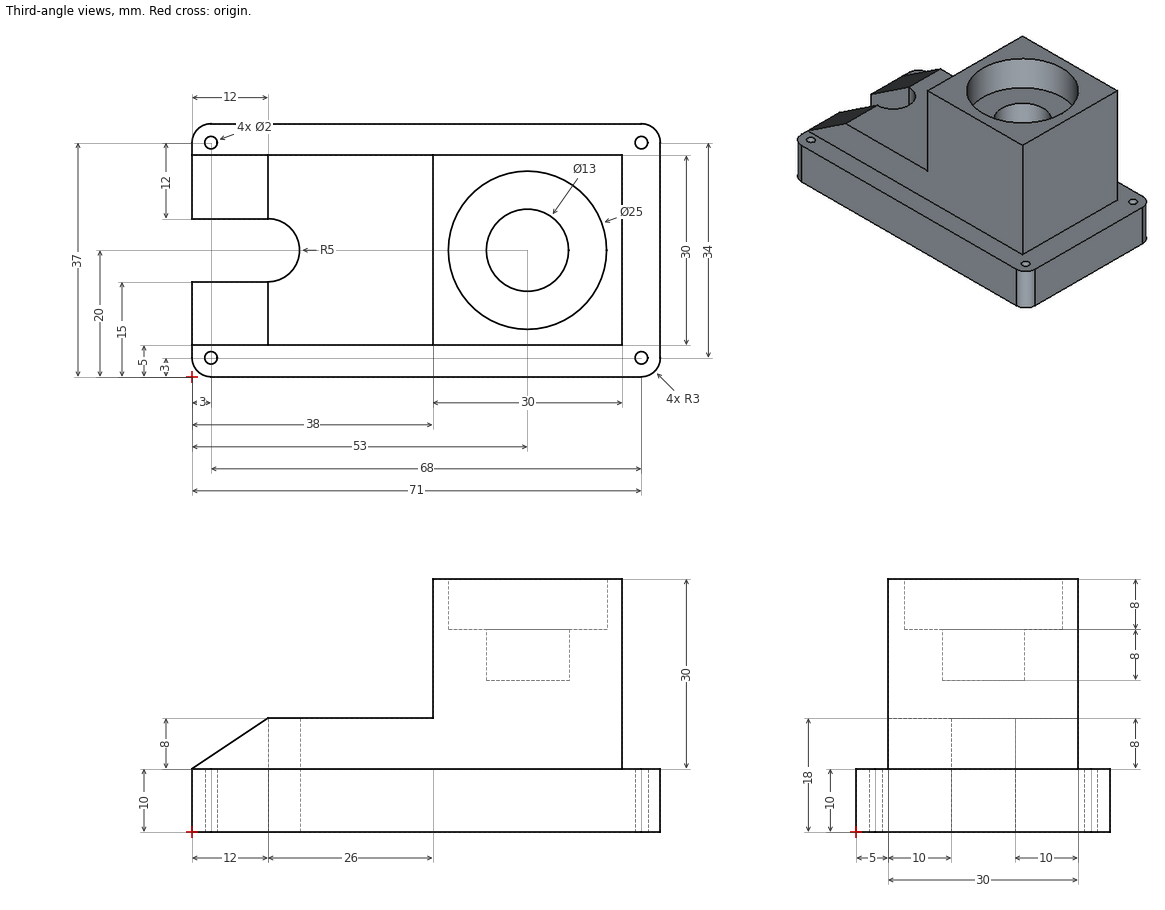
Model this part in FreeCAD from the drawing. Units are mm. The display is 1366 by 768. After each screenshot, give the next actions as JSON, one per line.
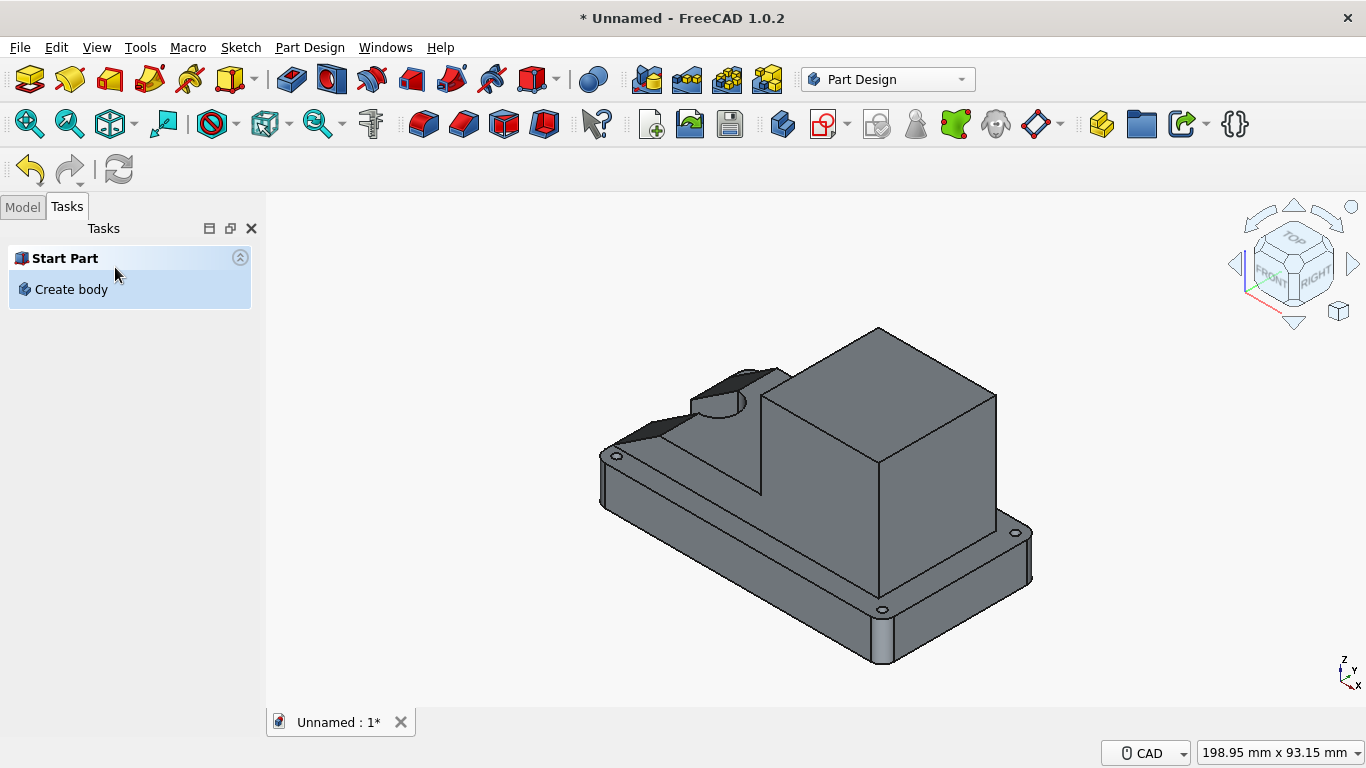
{"action": "left_click", "coordinate": [879, 394]}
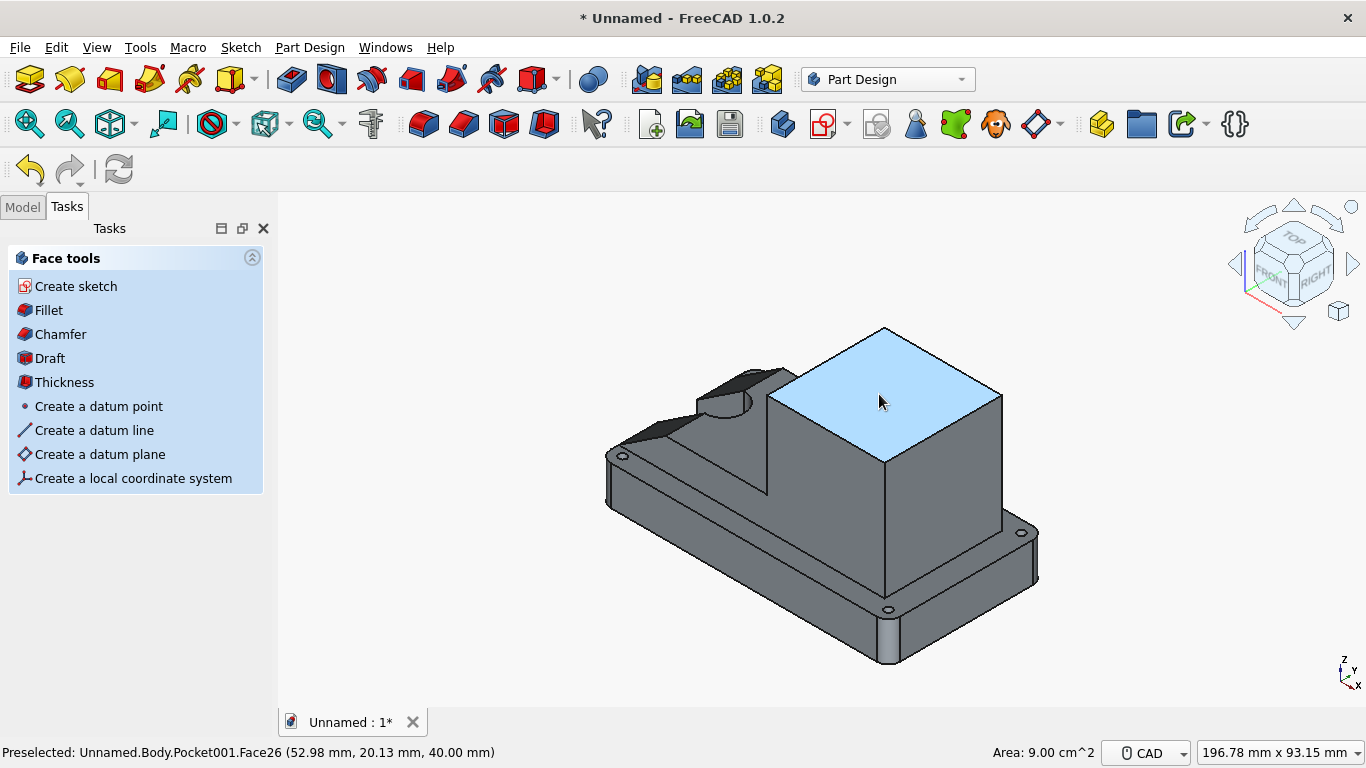
{"action": "left_click", "coordinate": [824, 124]}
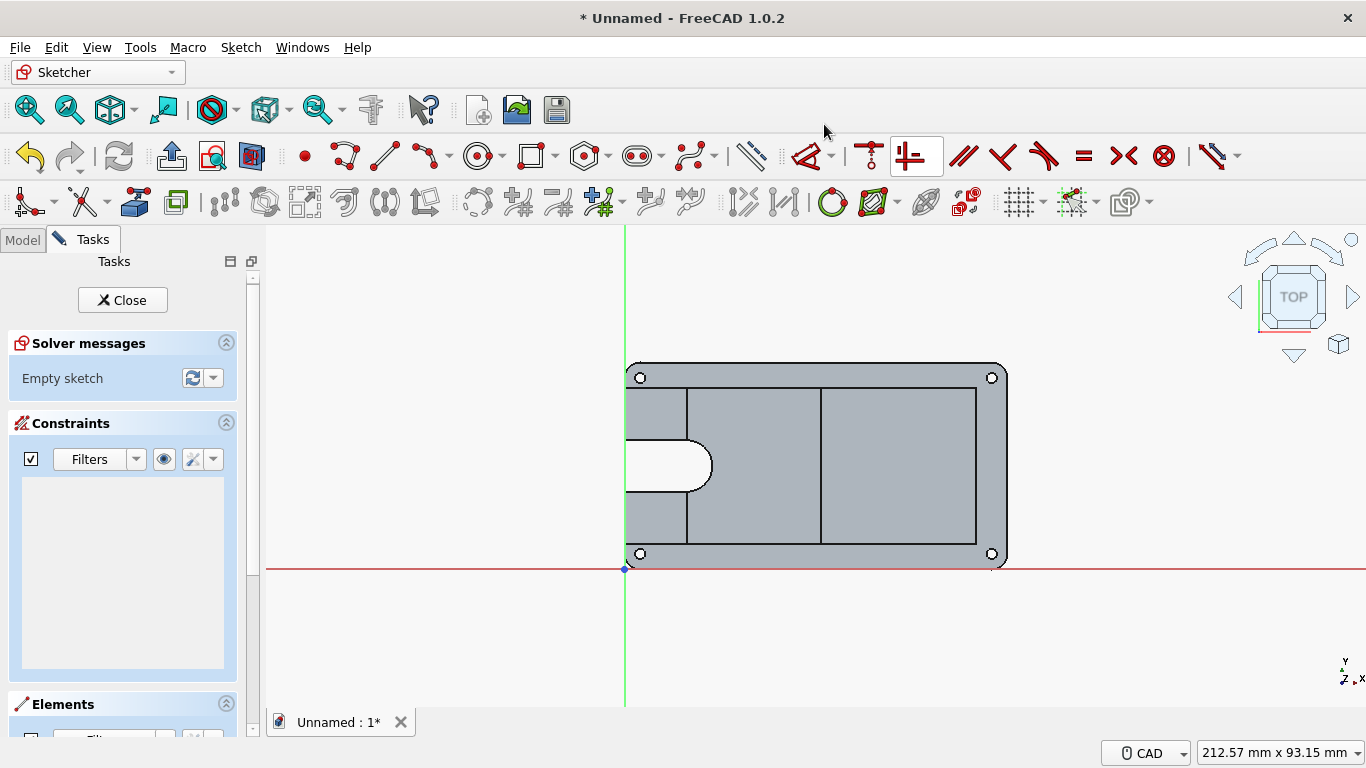
{"action": "scroll", "coordinate": [1022, 466], "scroll_direction": "up", "scroll_amount": 4}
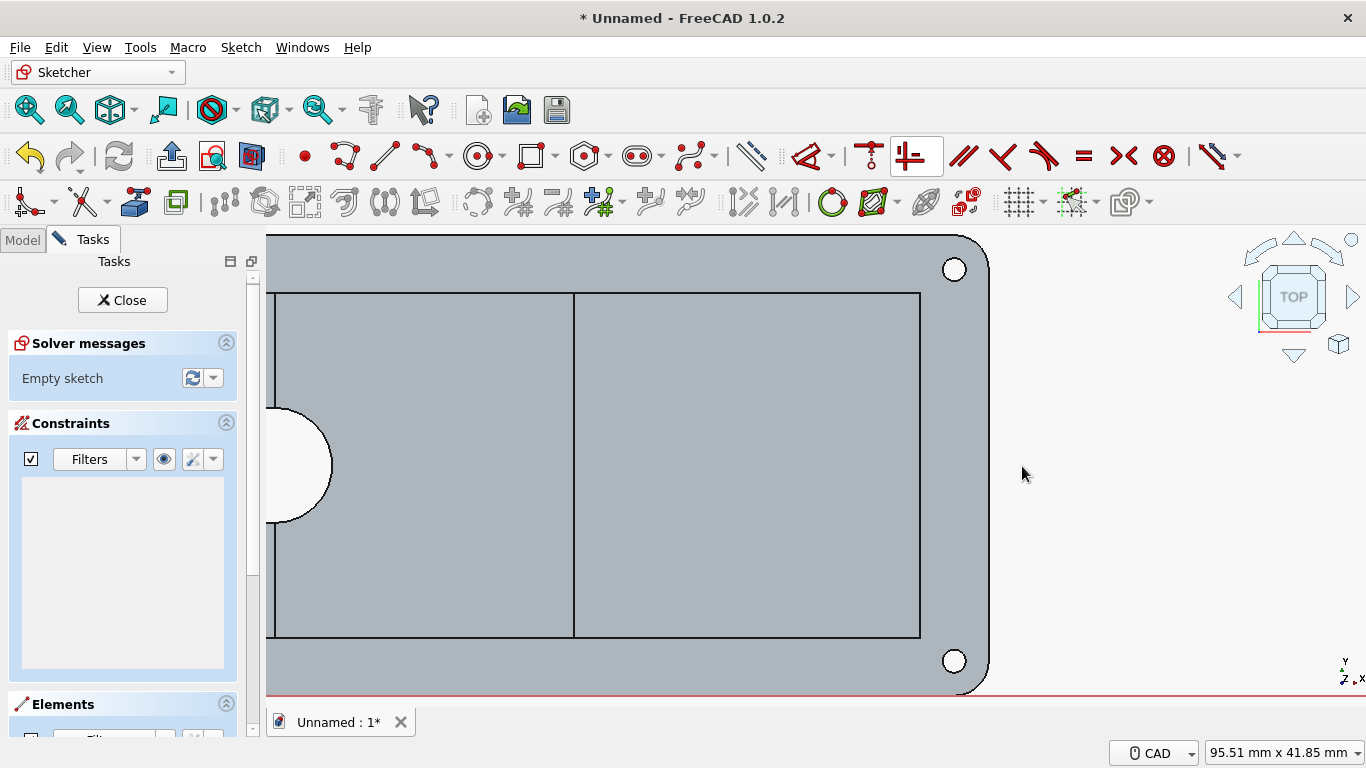
{"action": "left_click", "coordinate": [478, 156]}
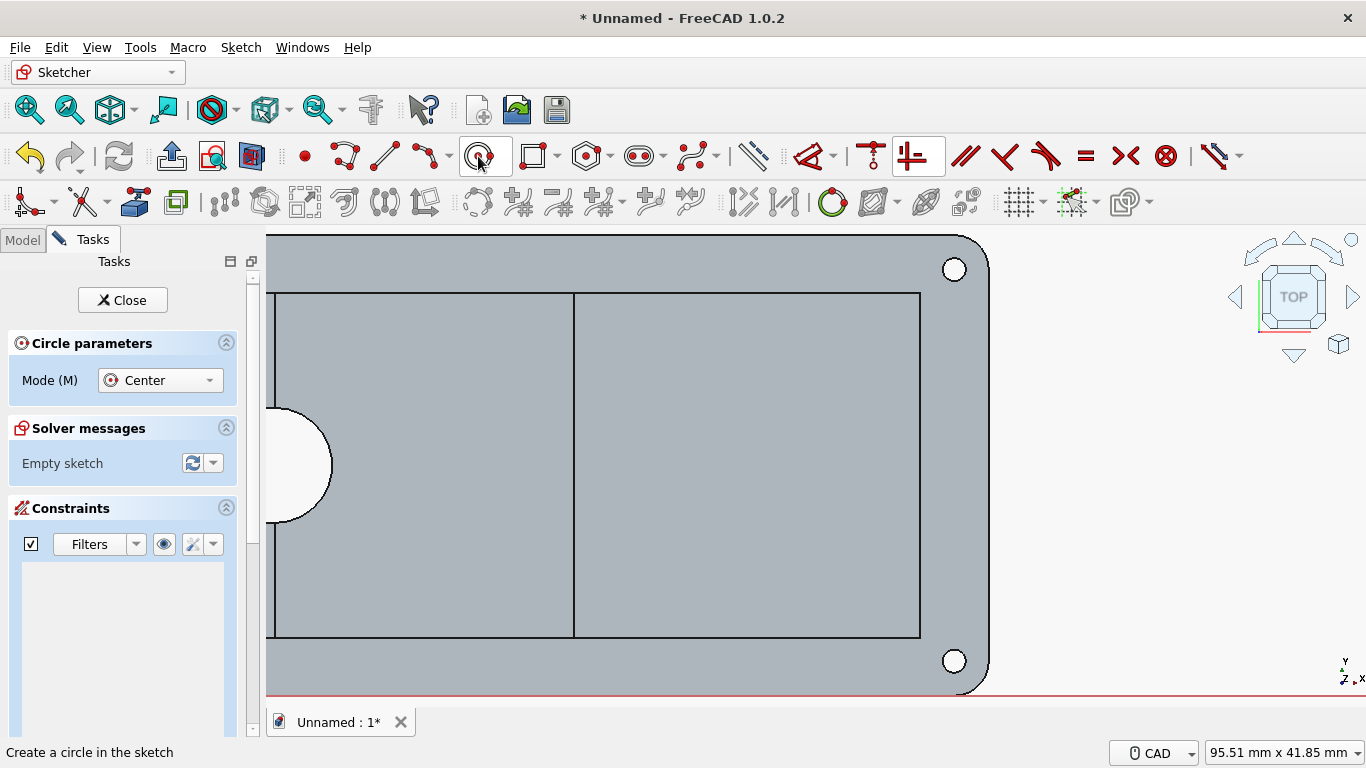
{"action": "left_click", "coordinate": [747, 465]}
{"action": "left_click", "coordinate": [849, 364]}
{"action": "key", "text": "Escape"}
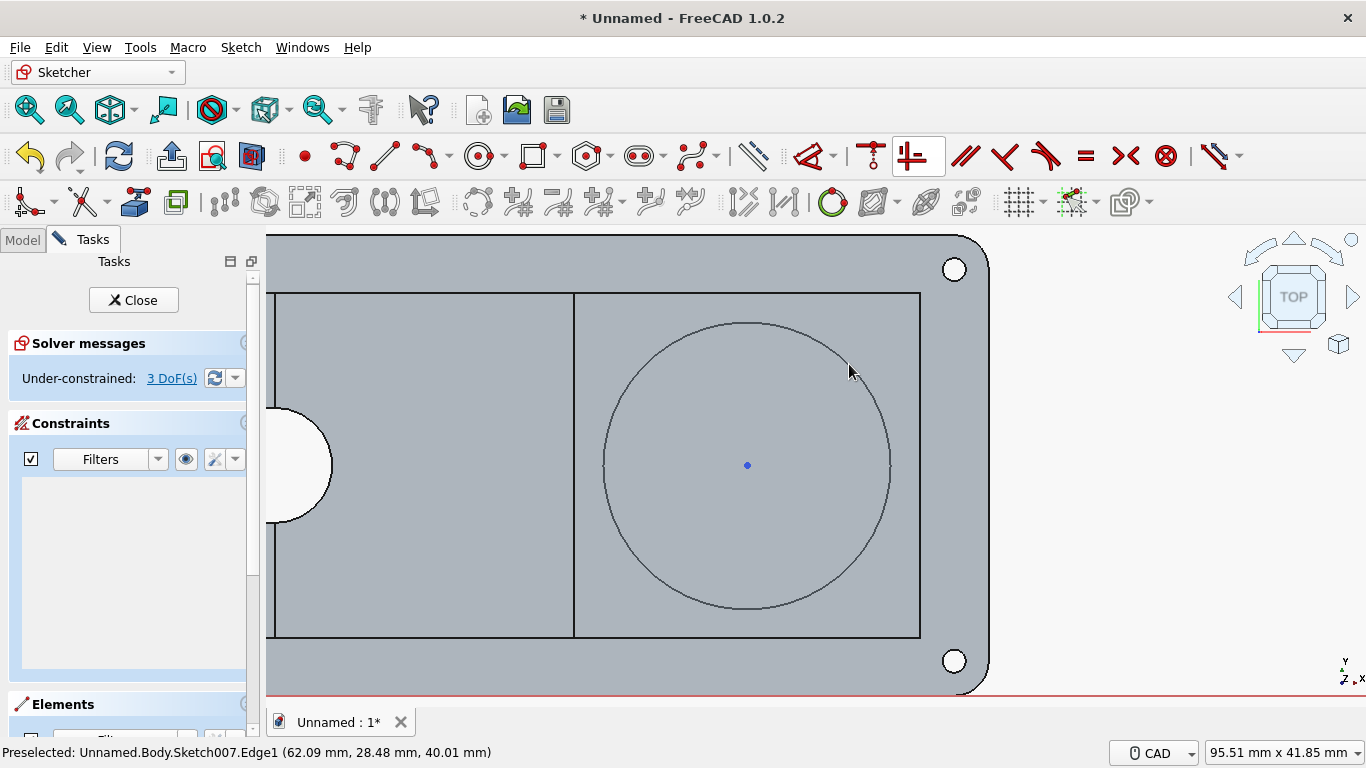
{"action": "left_click", "coordinate": [808, 156]}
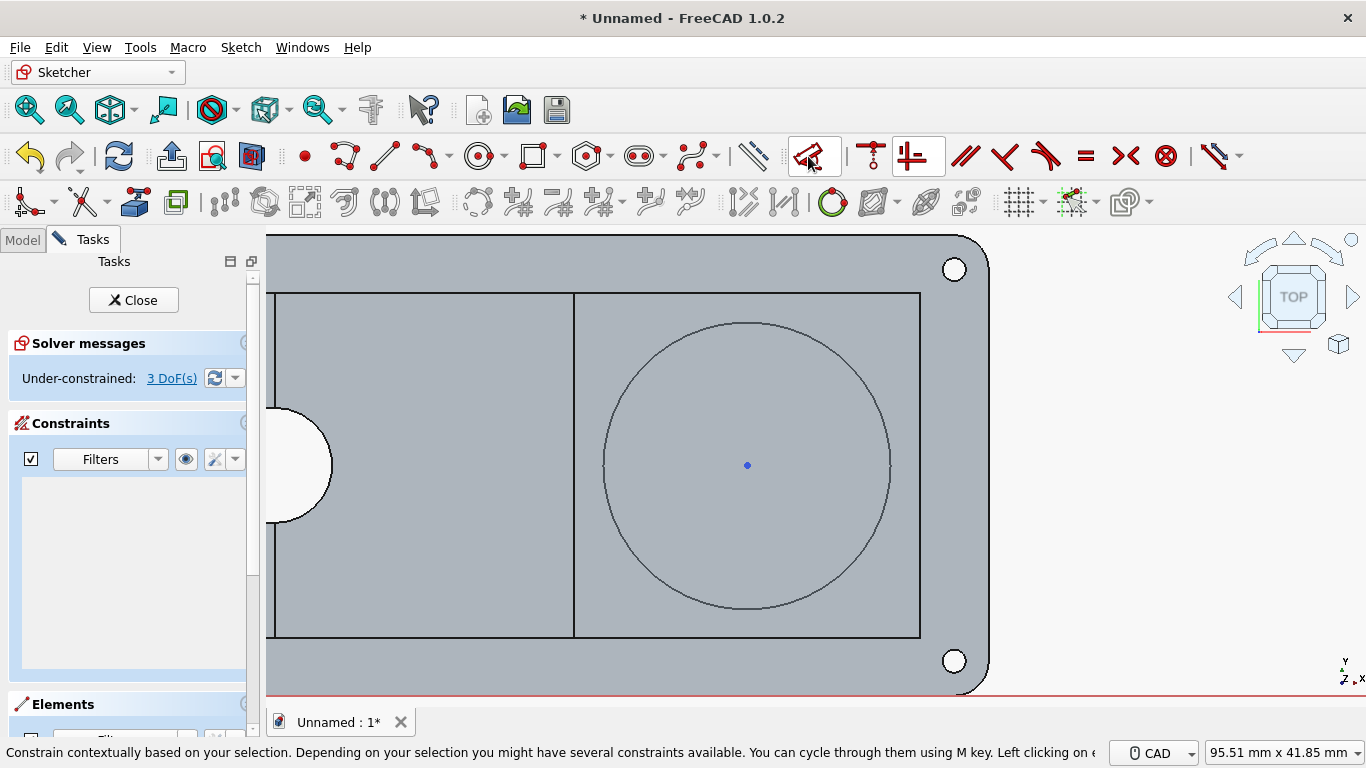
{"action": "left_click", "coordinate": [848, 364]}
{"action": "left_click", "coordinate": [871, 341]}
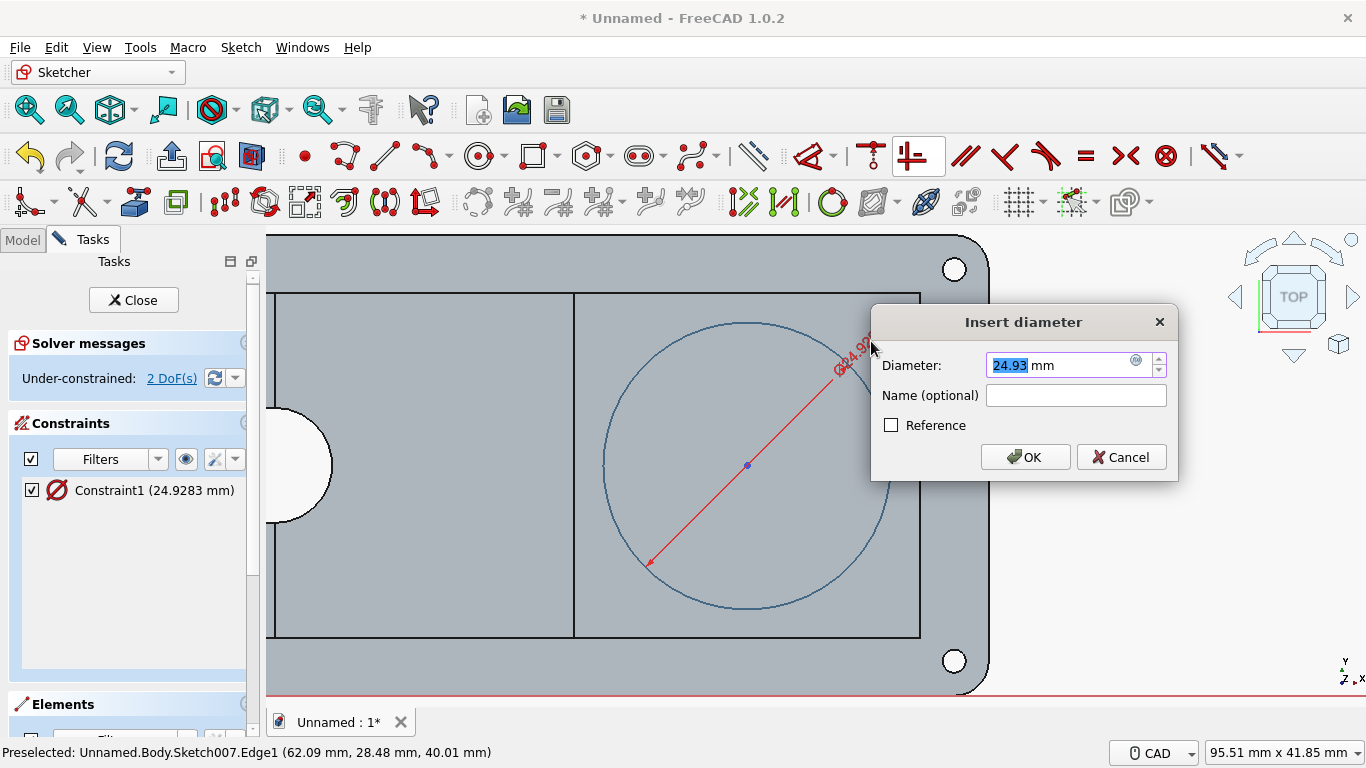
{"action": "type", "text": "25"}
{"action": "key", "text": "Return"}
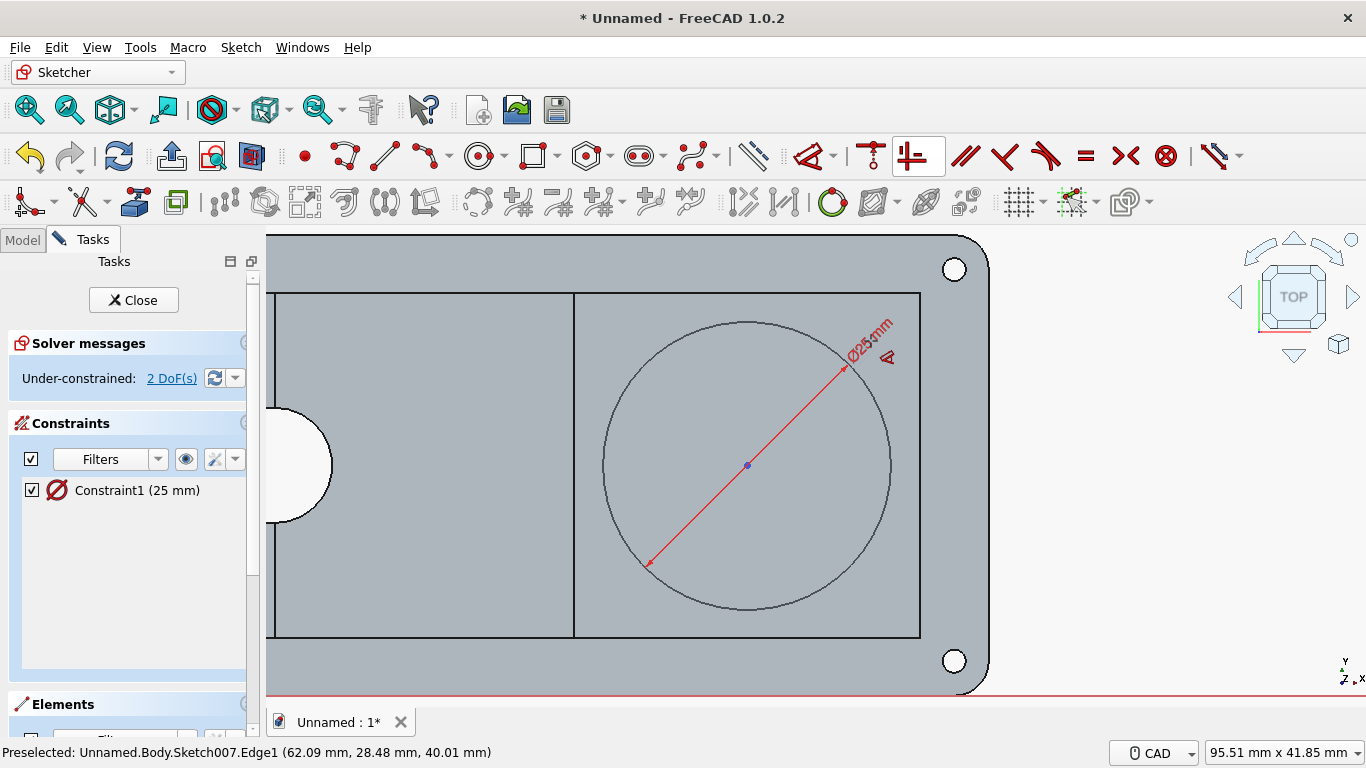
{"action": "left_click", "coordinate": [747, 466]}
{"action": "left_click", "coordinate": [521, 432]}